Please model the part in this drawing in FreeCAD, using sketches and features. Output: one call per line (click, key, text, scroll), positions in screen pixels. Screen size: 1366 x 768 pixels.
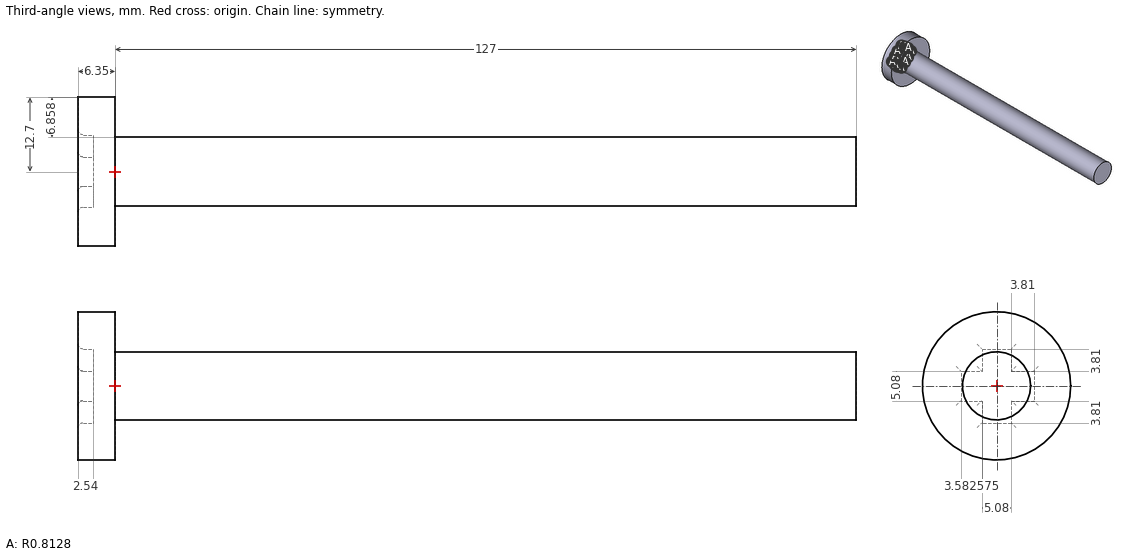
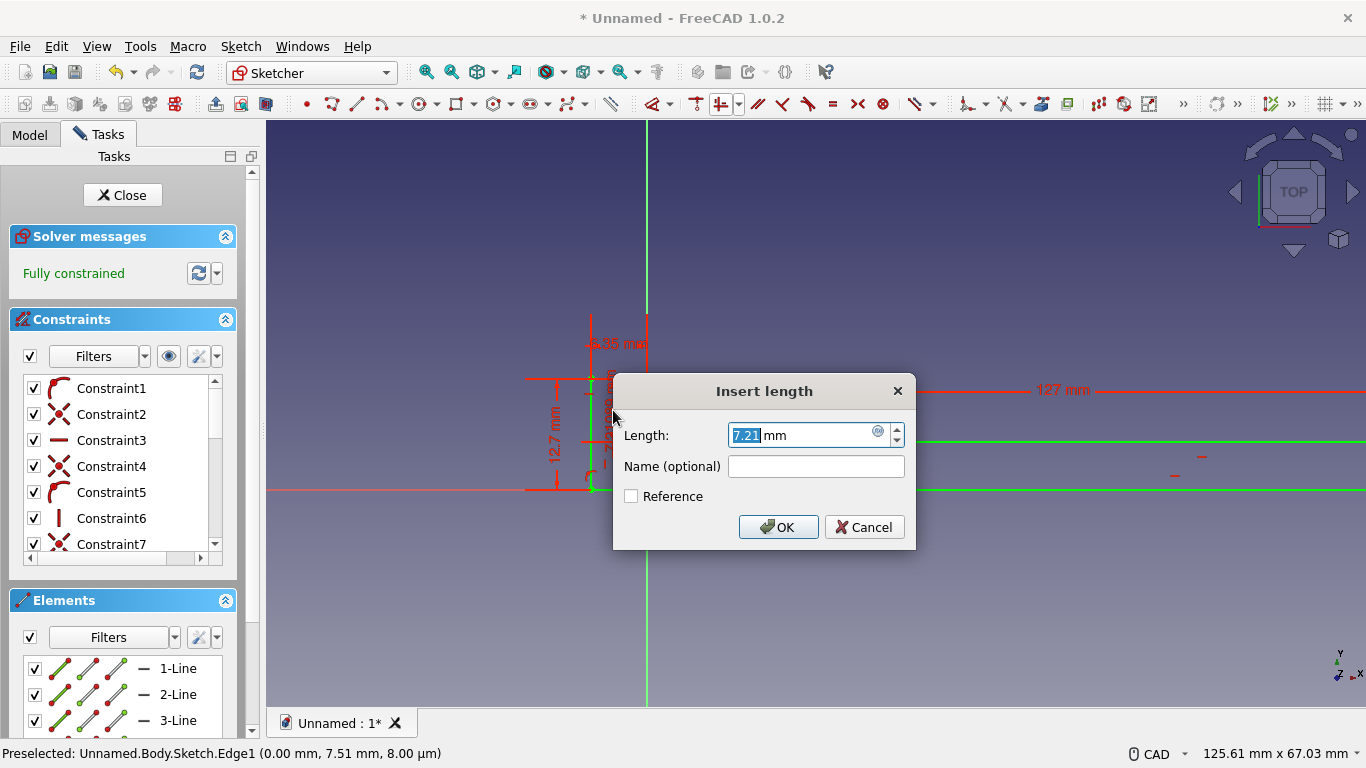
text(6.858)
key(Return)
key(Escape)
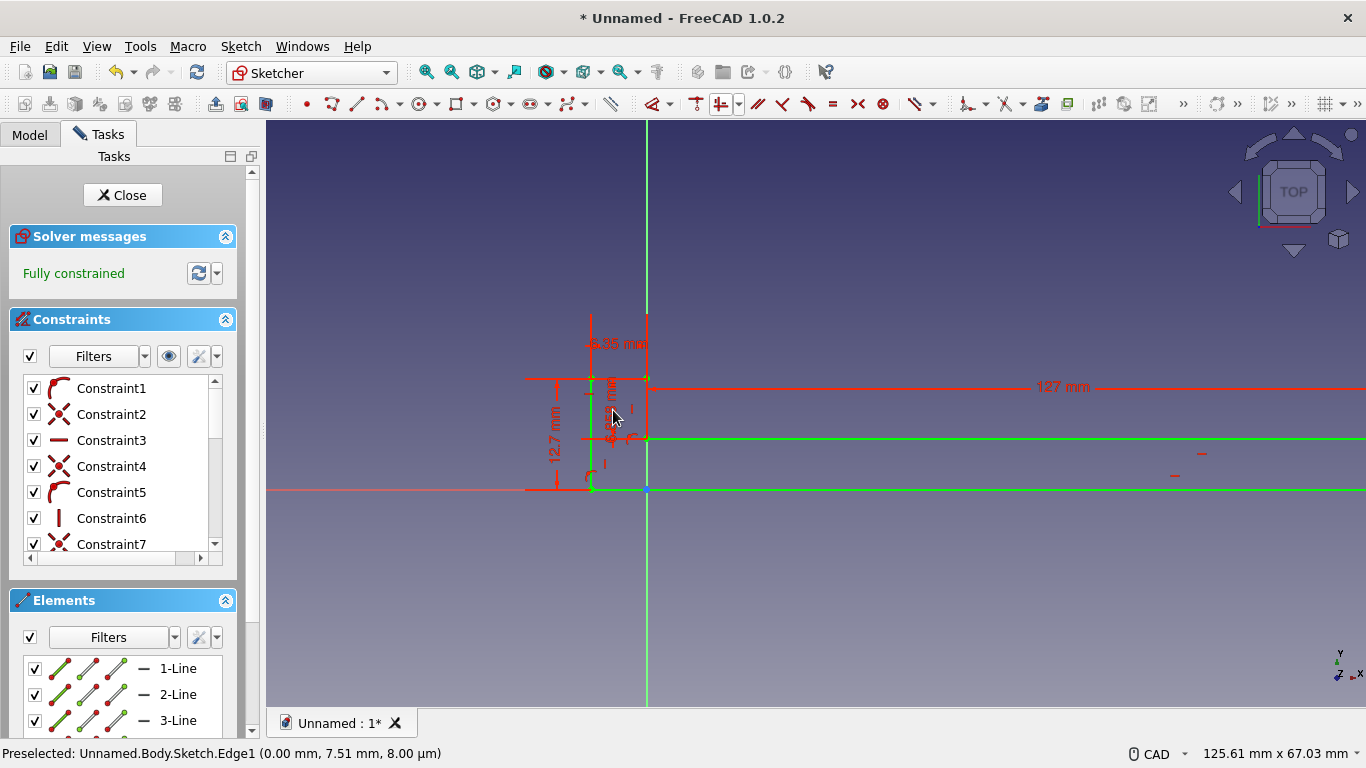
click(123, 195)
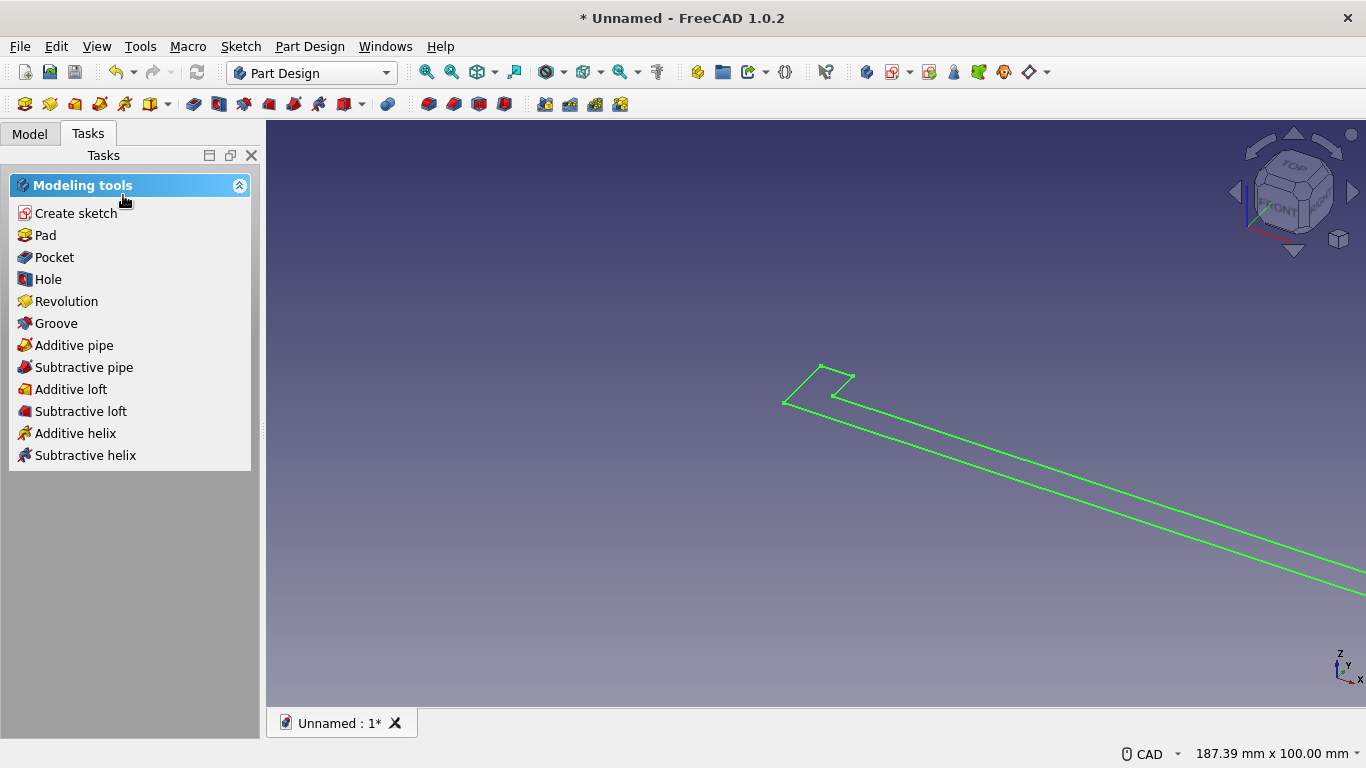
click(50, 104)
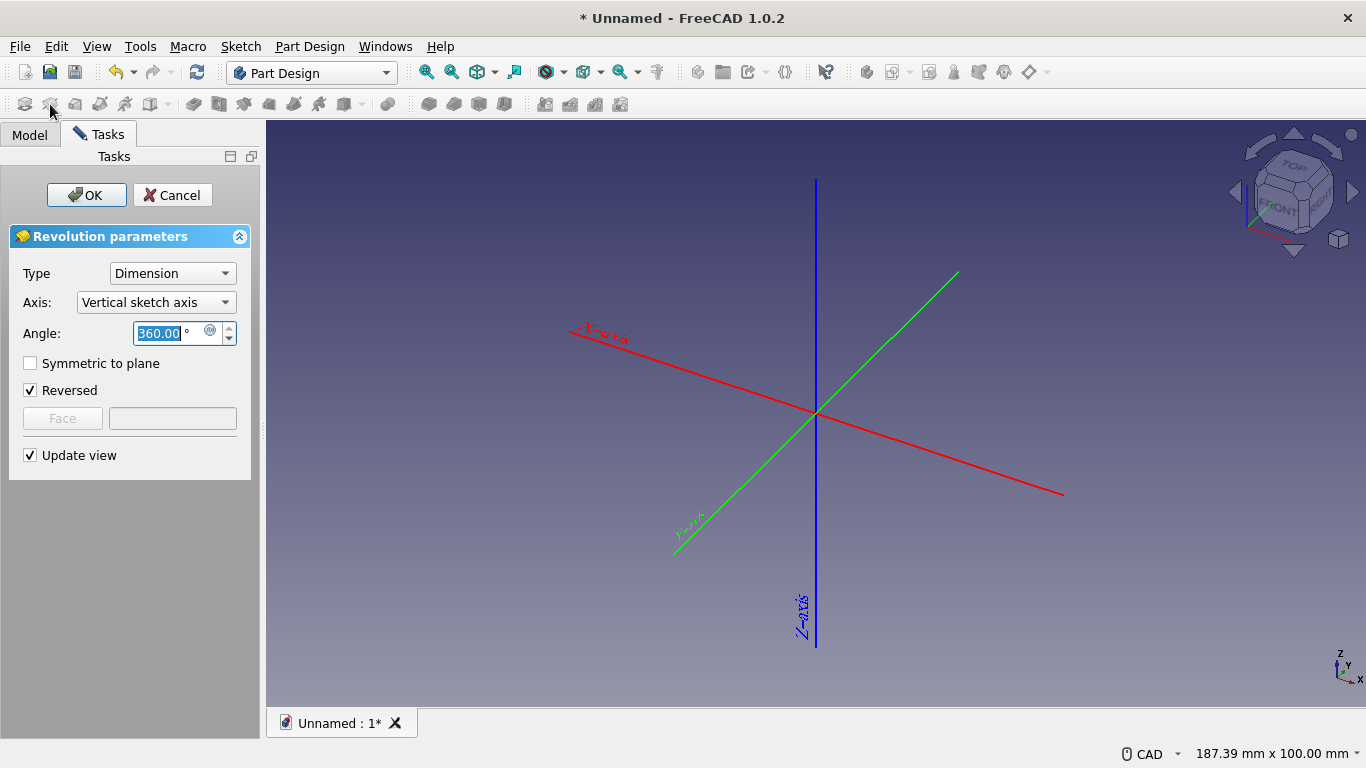
click(157, 302)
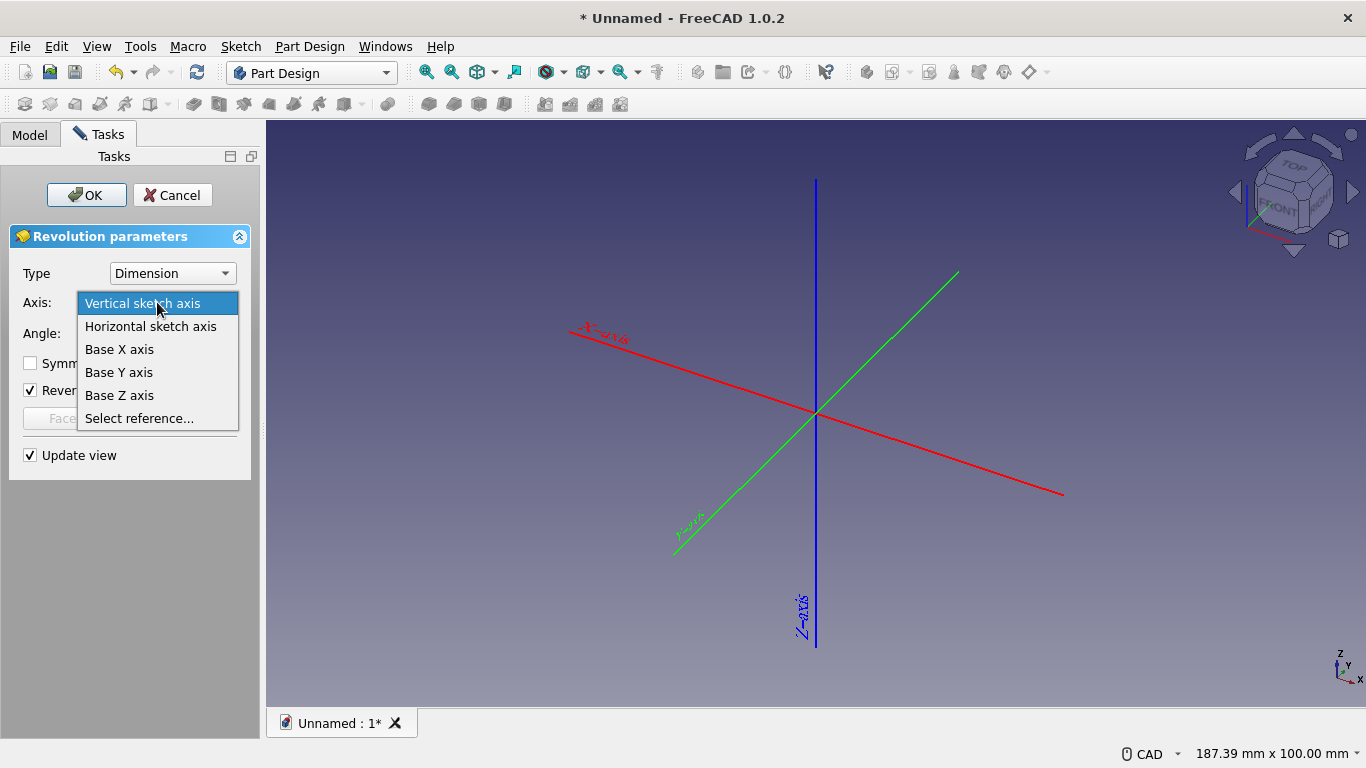
click(156, 326)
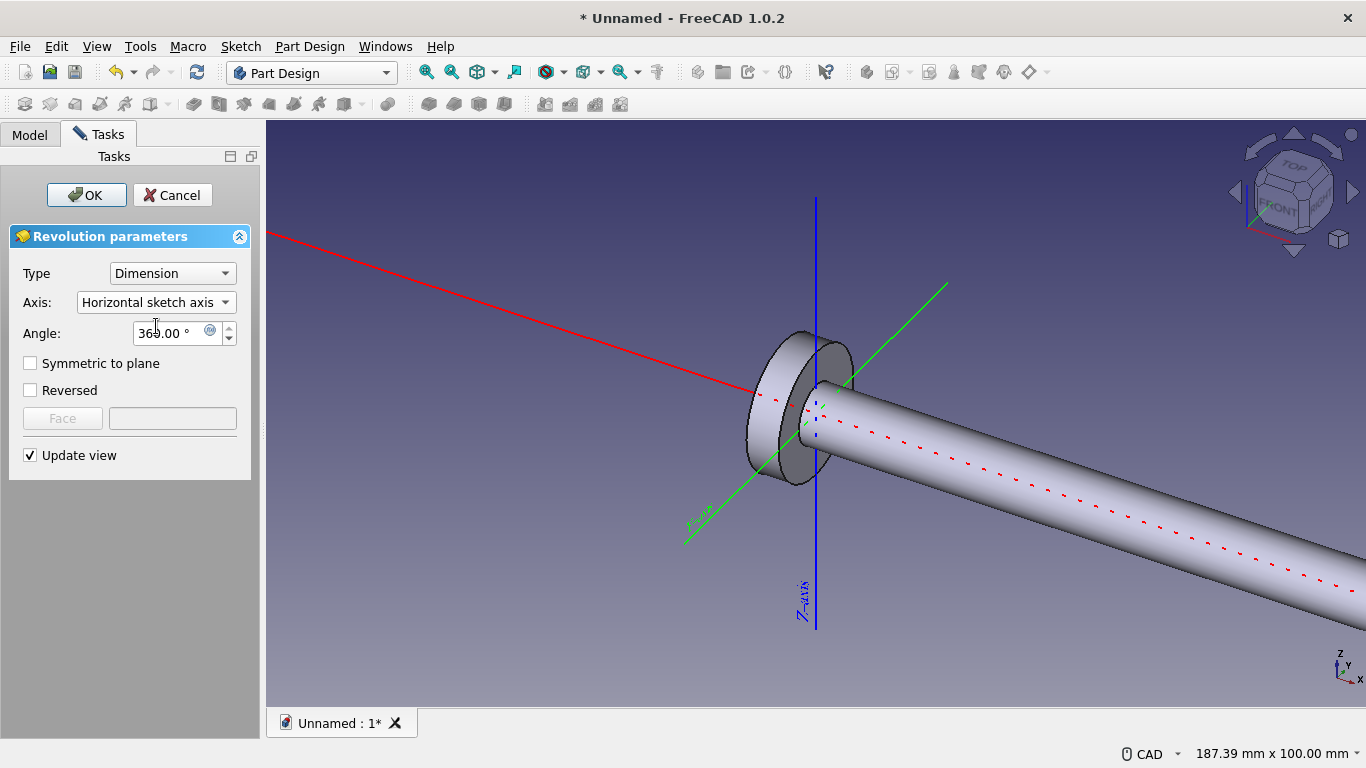
click(87, 195)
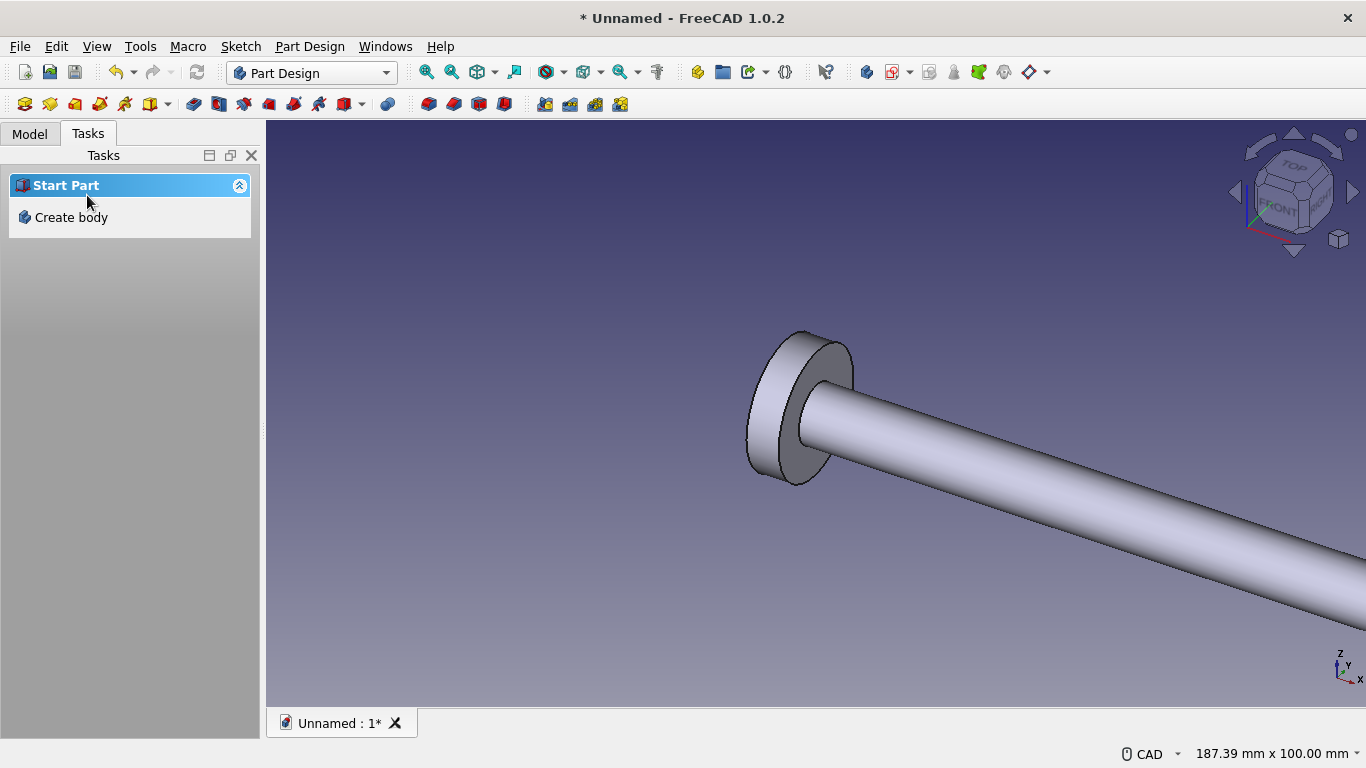
click(427, 72)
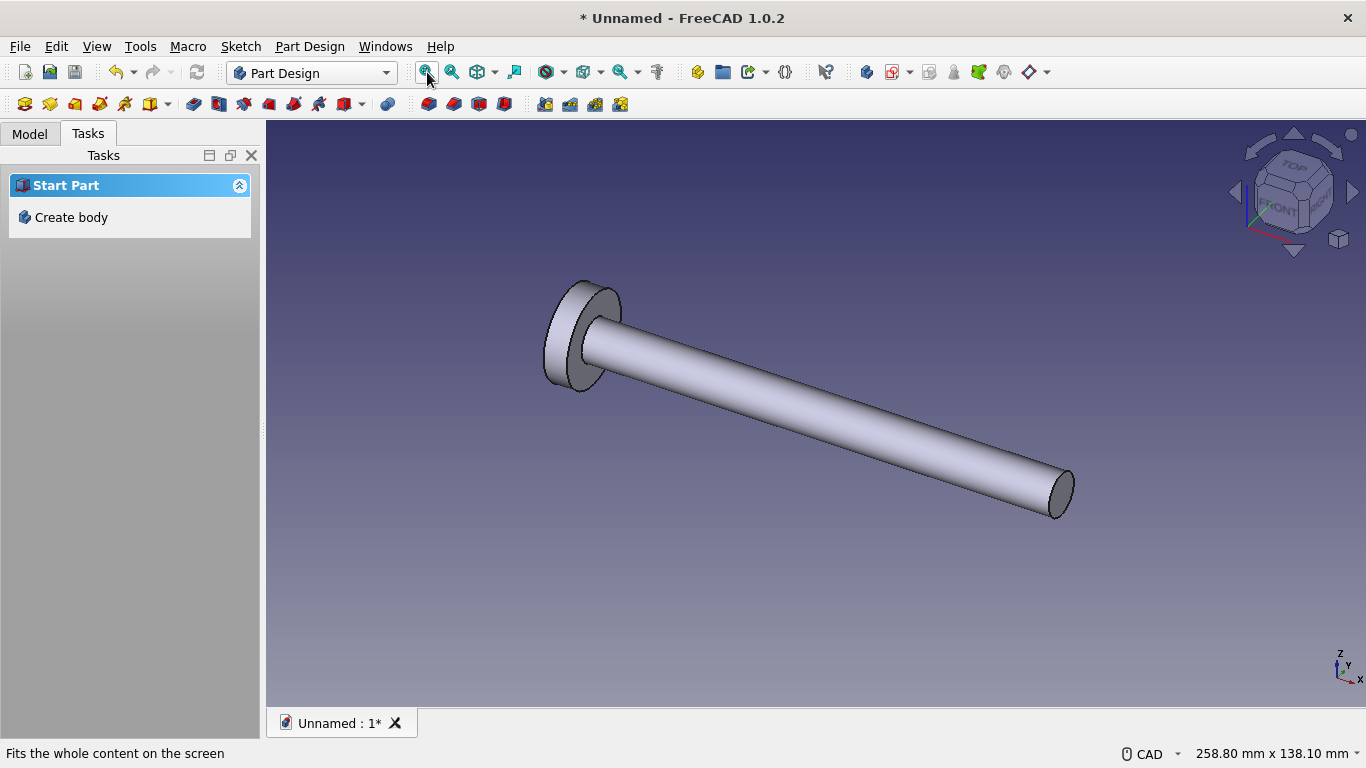
key(6)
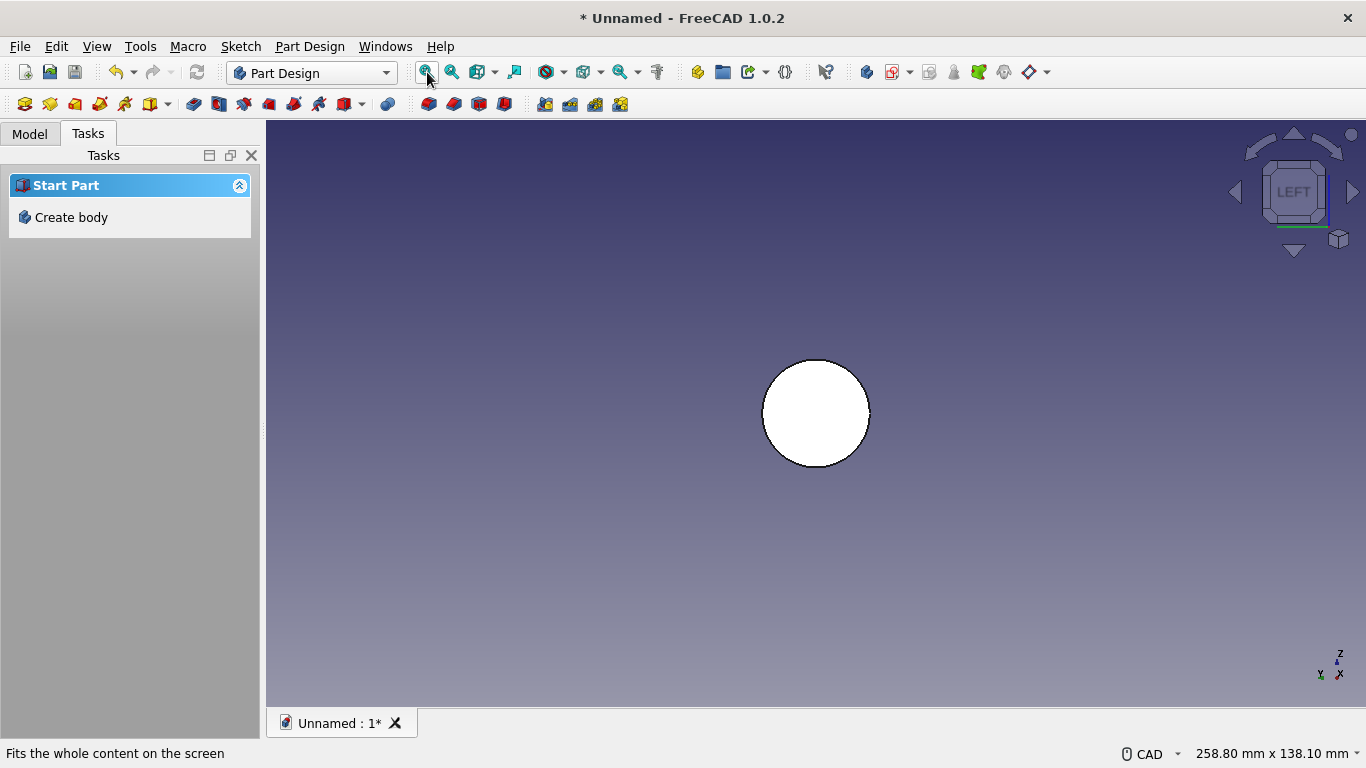
click(427, 72)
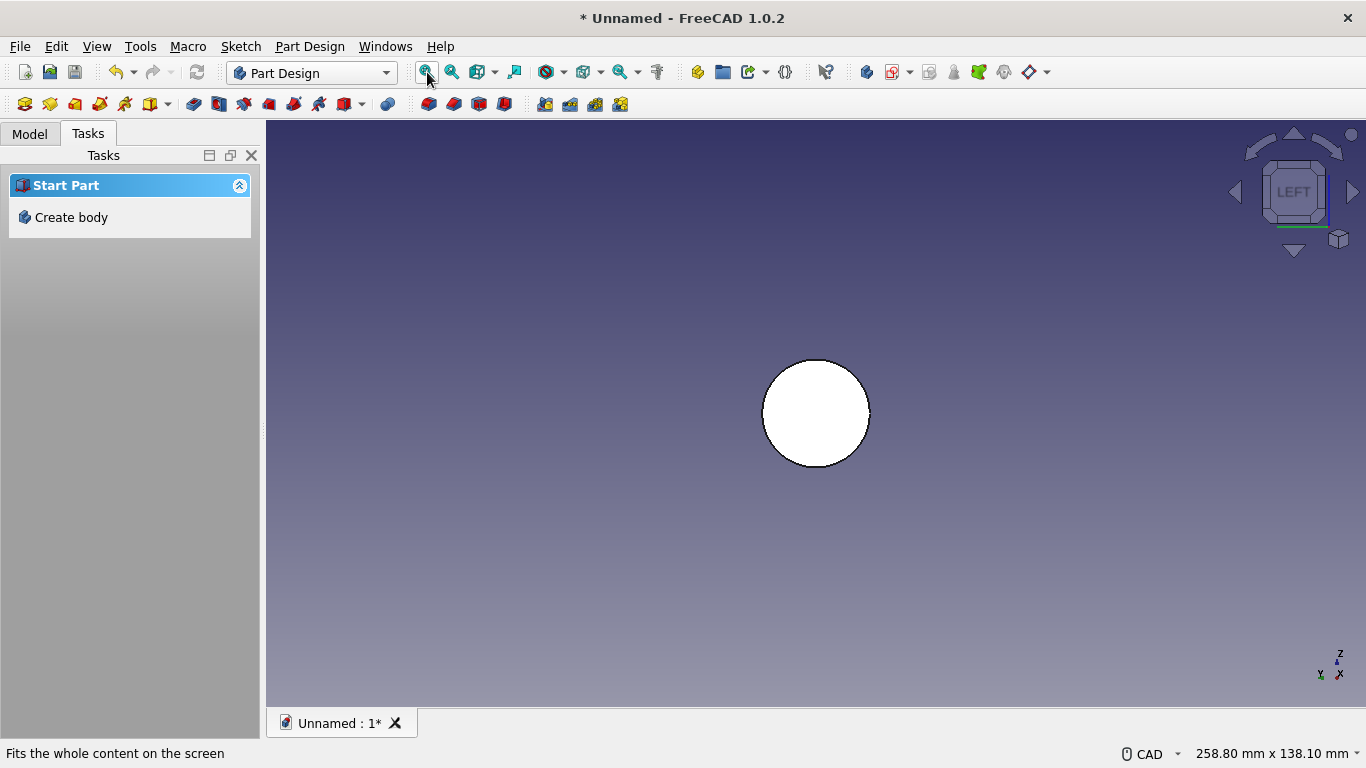
click(816, 412)